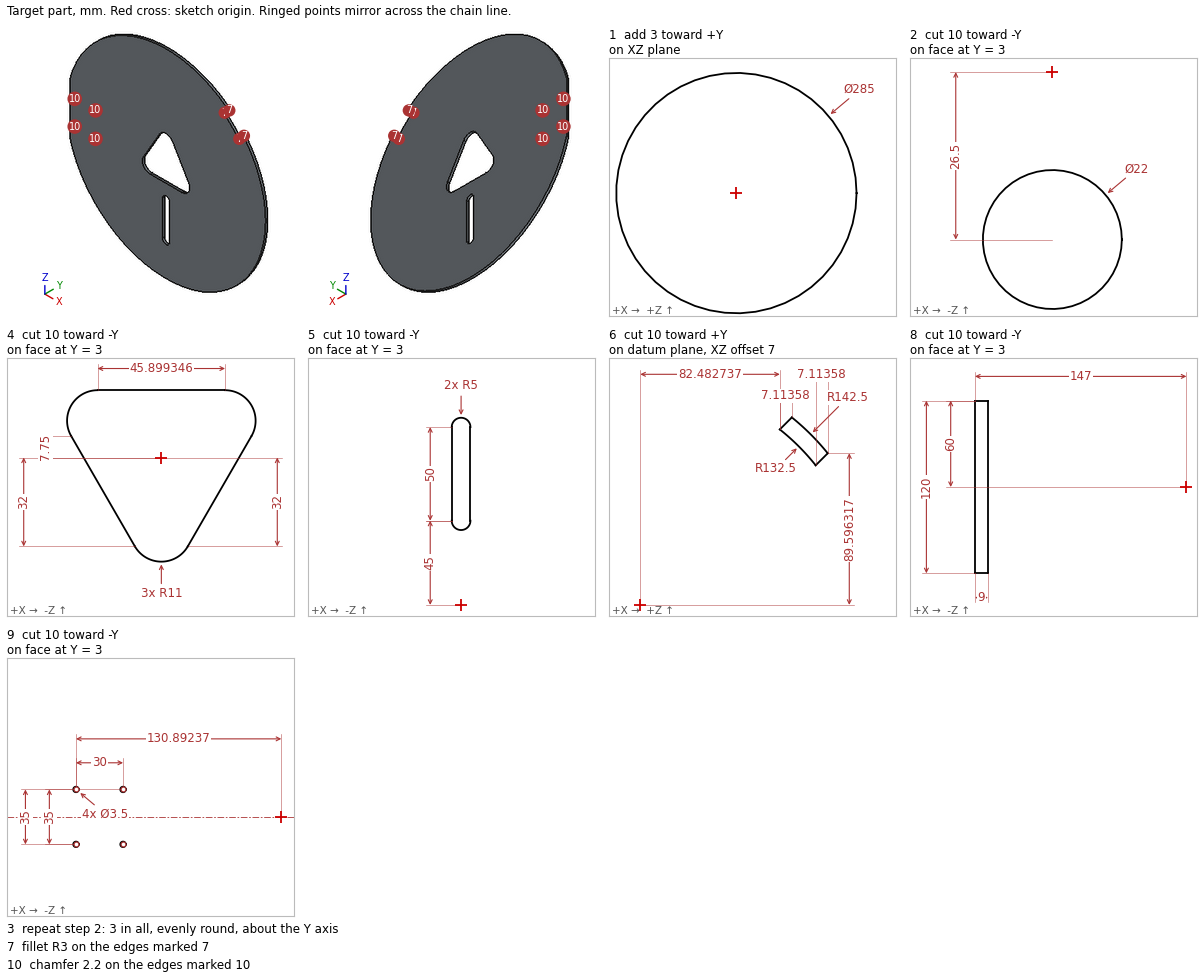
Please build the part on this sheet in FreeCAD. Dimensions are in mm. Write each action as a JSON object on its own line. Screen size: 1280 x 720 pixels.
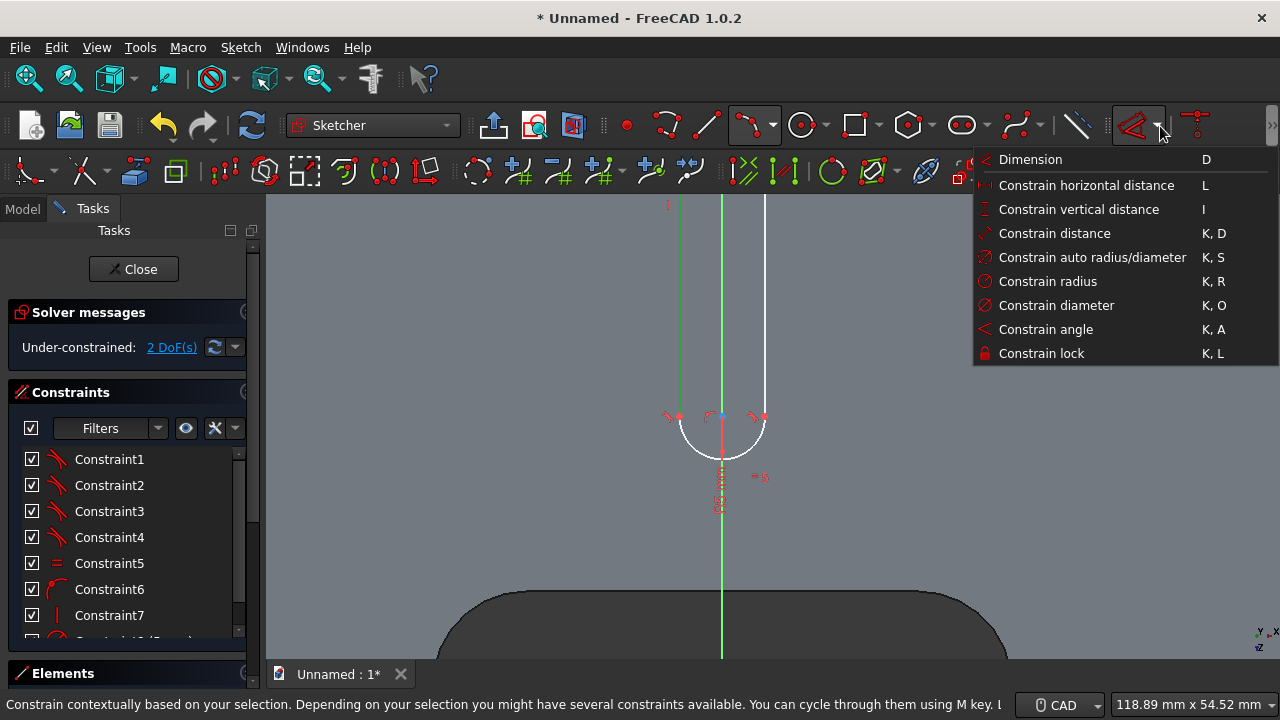
{"action": "left_click", "coordinate": [1126, 209]}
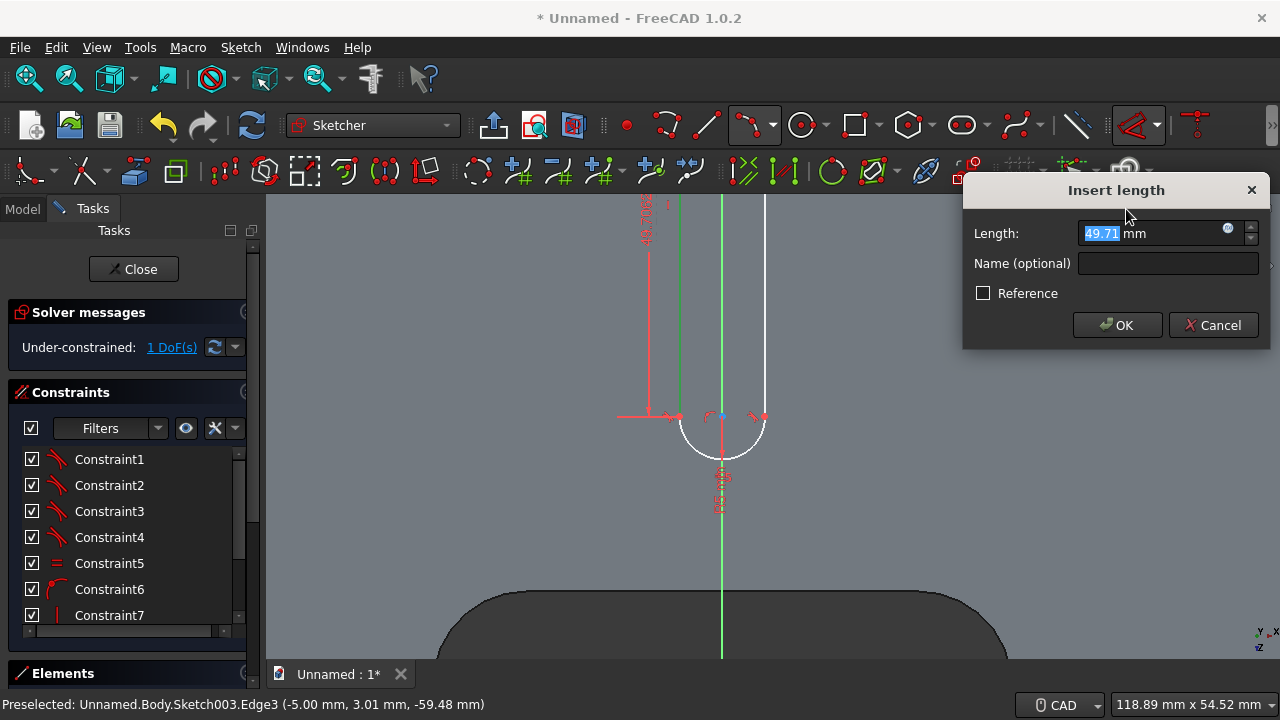
{"action": "type", "text": "50"}
{"action": "key", "text": "Return"}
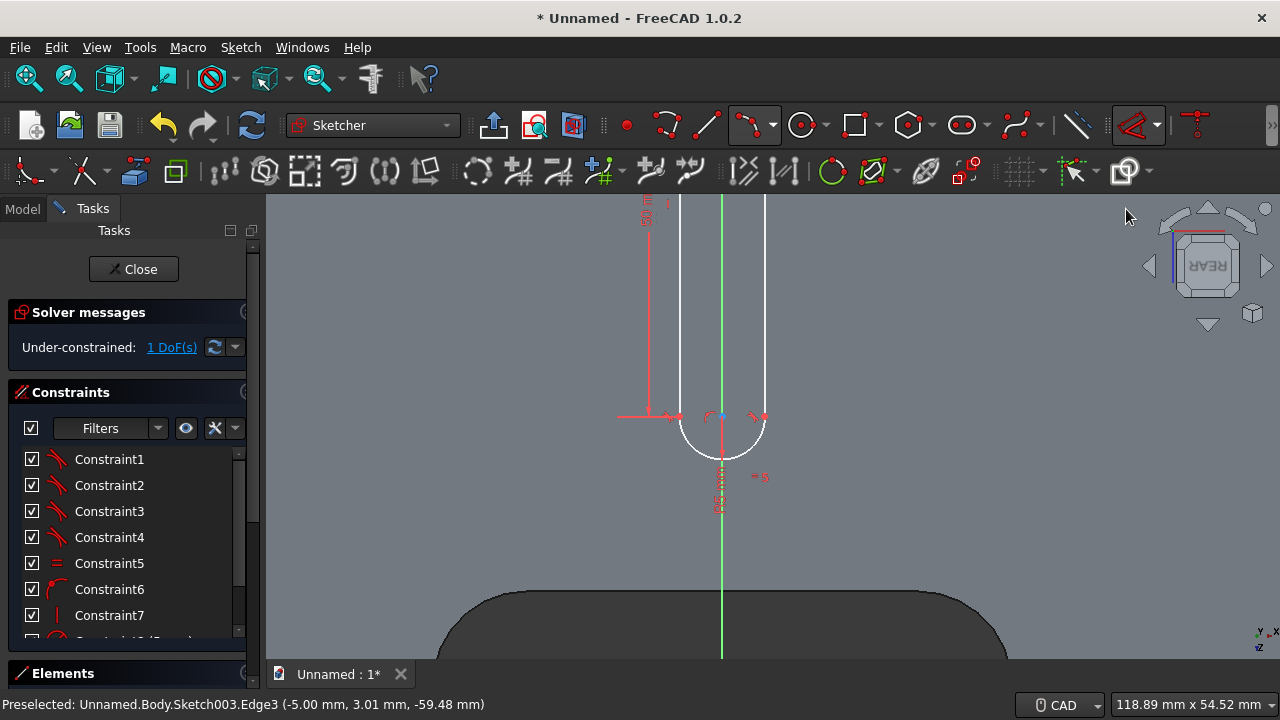
{"action": "left_click", "coordinate": [680, 417]}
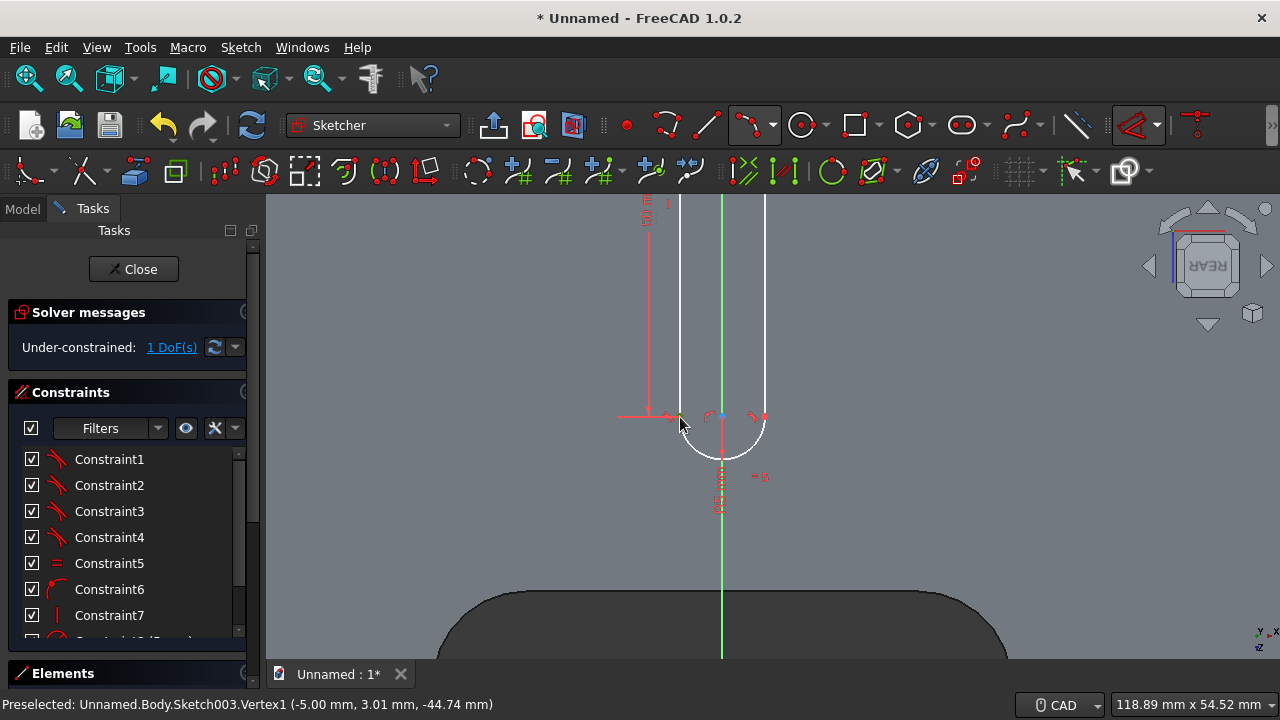
{"action": "key", "text": "i"}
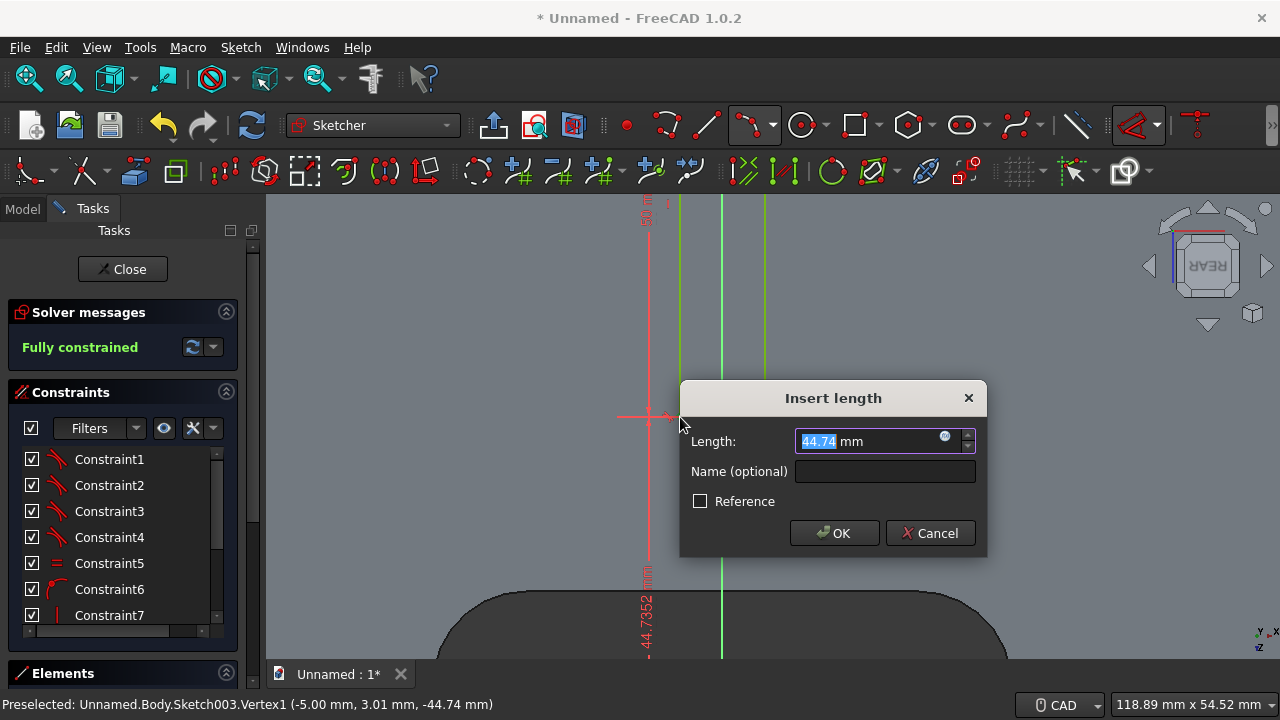
{"action": "type", "text": "45"}
{"action": "key", "text": "Return"}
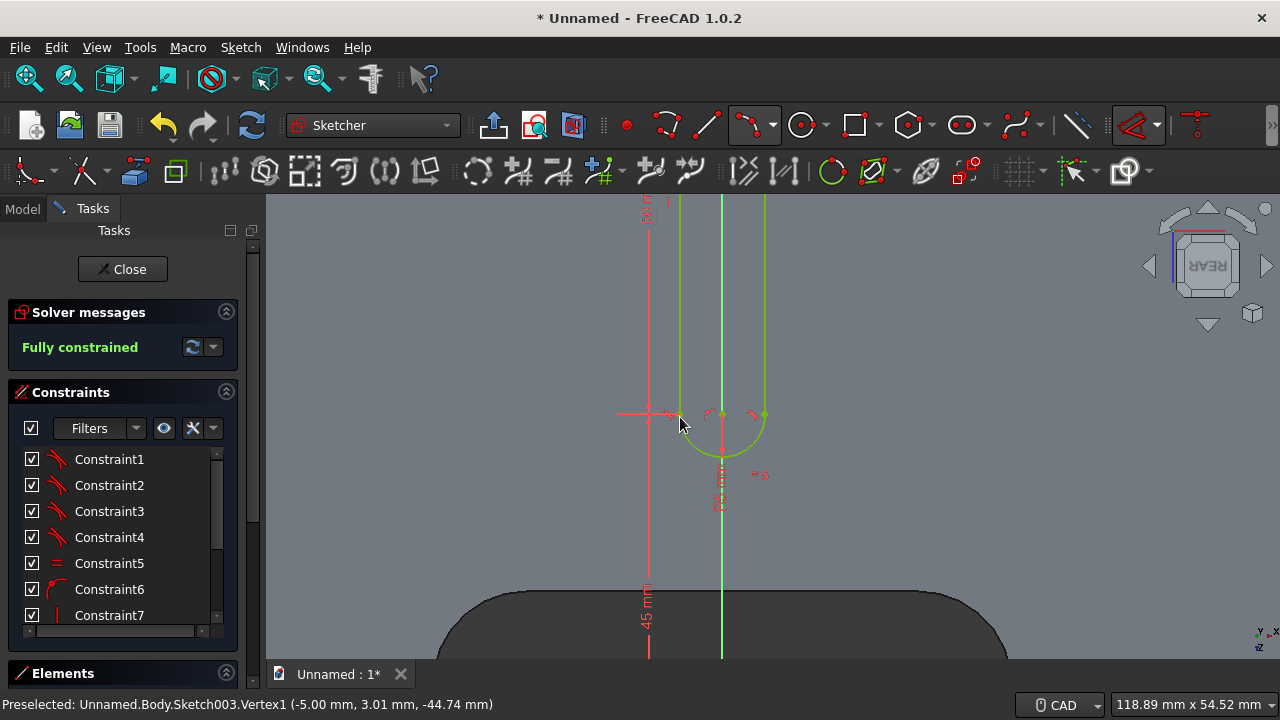
{"action": "left_click", "coordinate": [123, 269]}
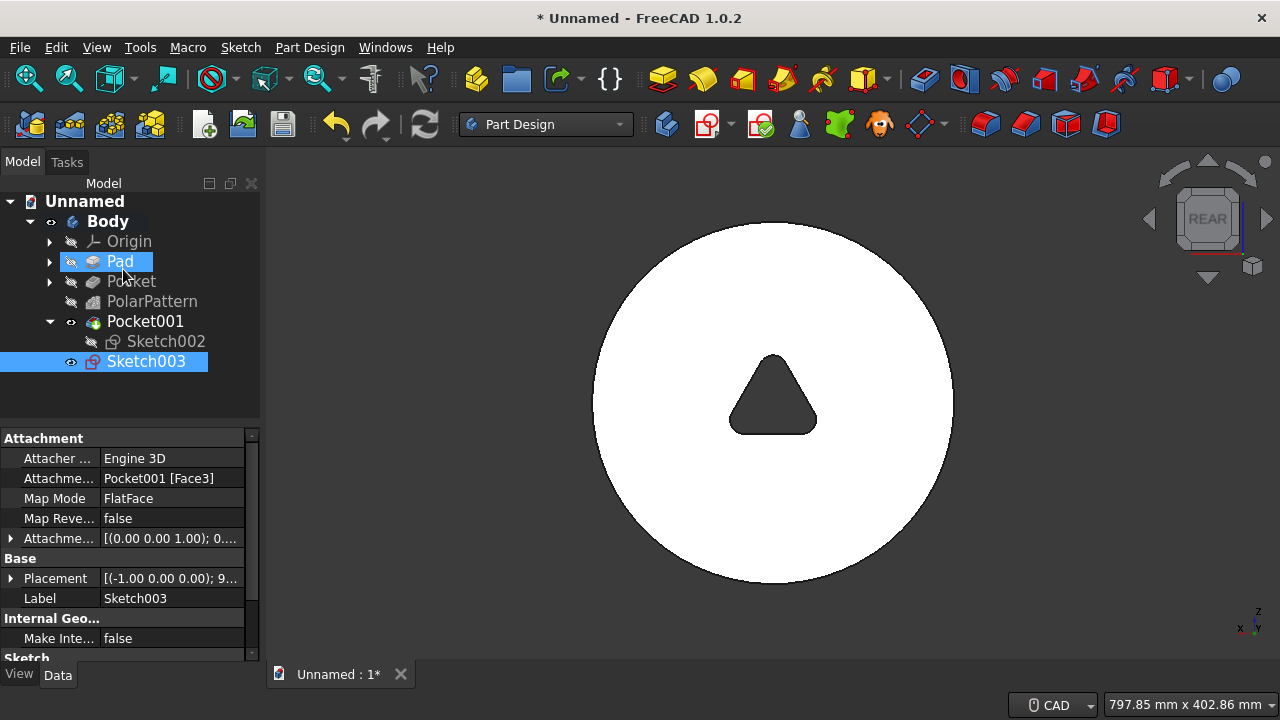
{"action": "left_click", "coordinate": [926, 80]}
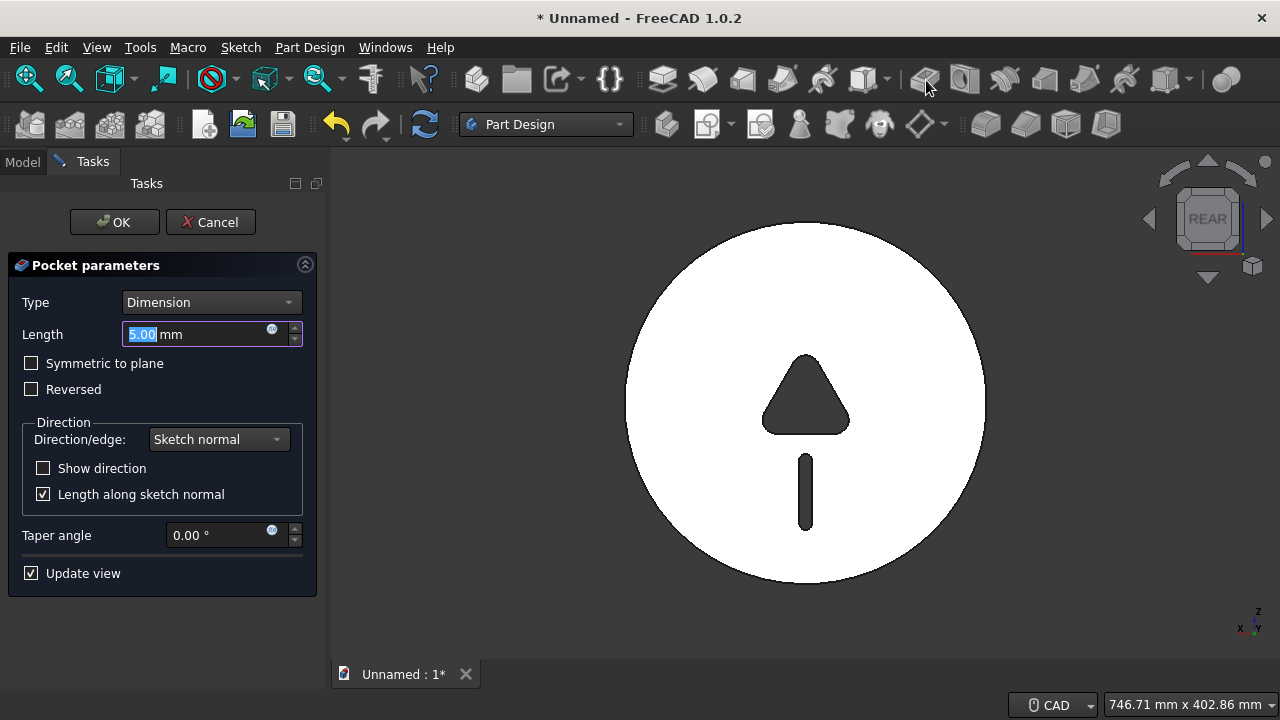
{"action": "type", "text": "10"}
{"action": "key", "text": "Tab"}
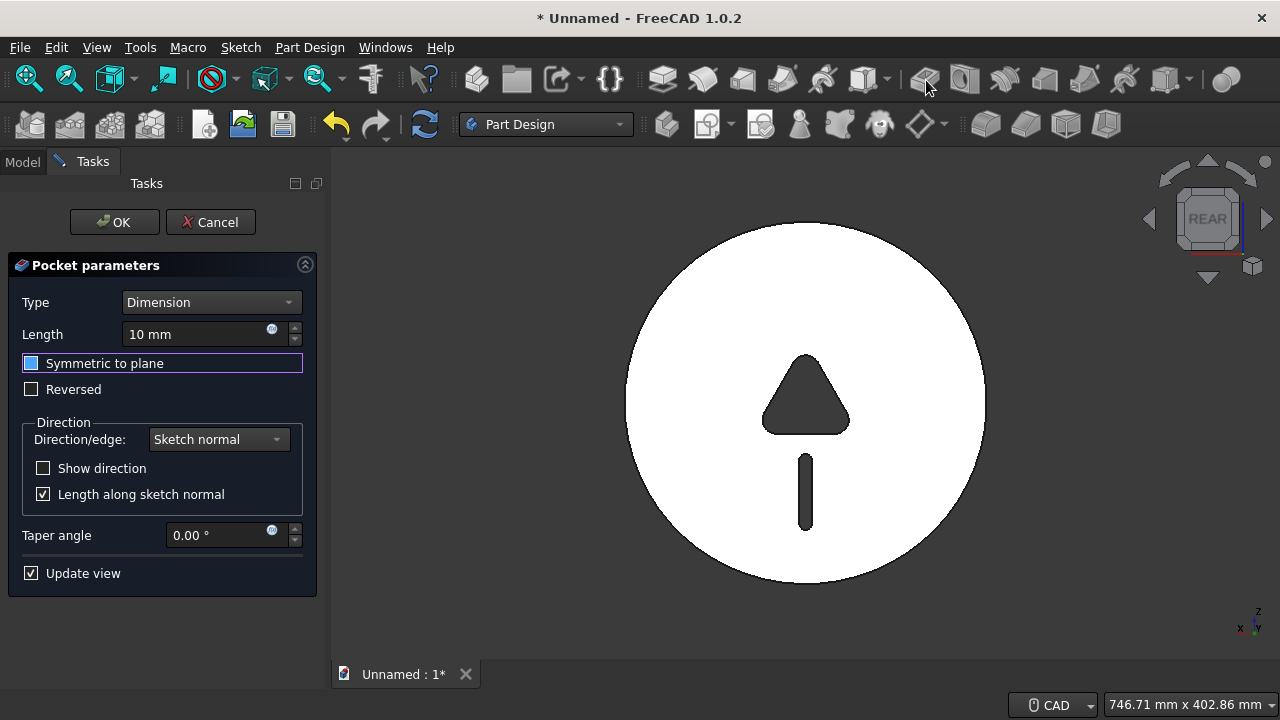
{"action": "left_click", "coordinate": [115, 222]}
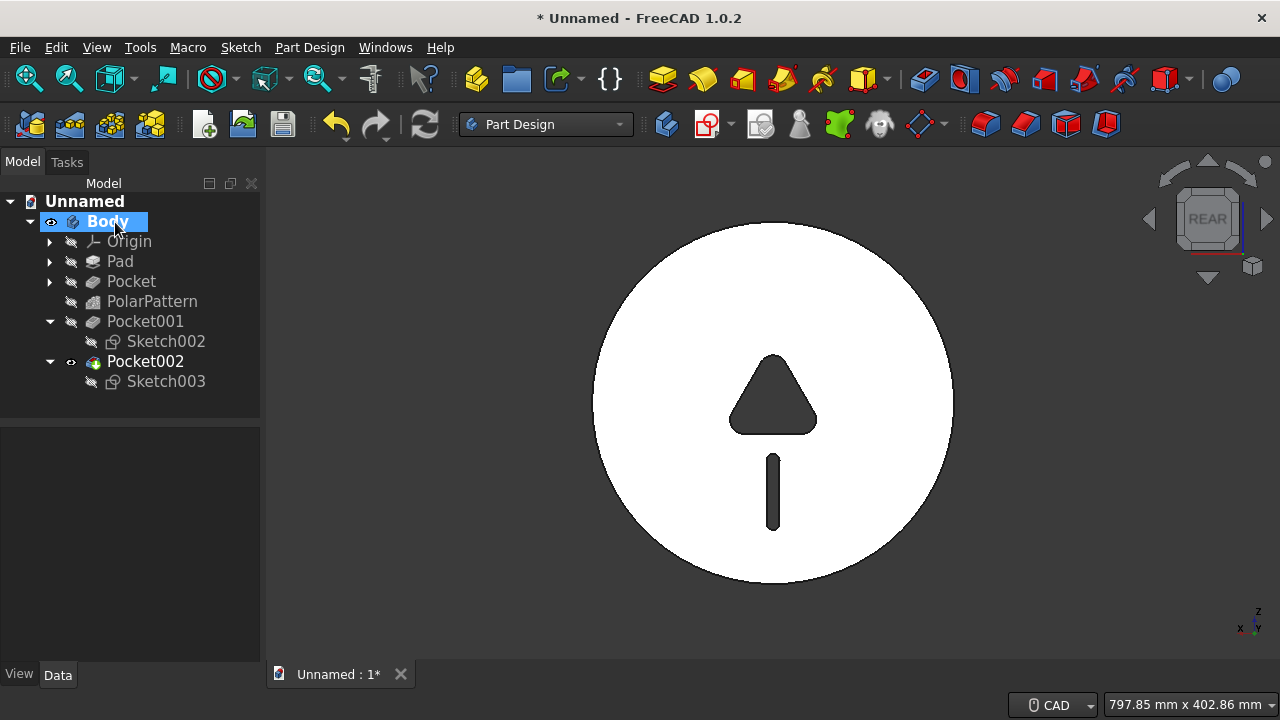
{"action": "left_click", "coordinate": [50, 242]}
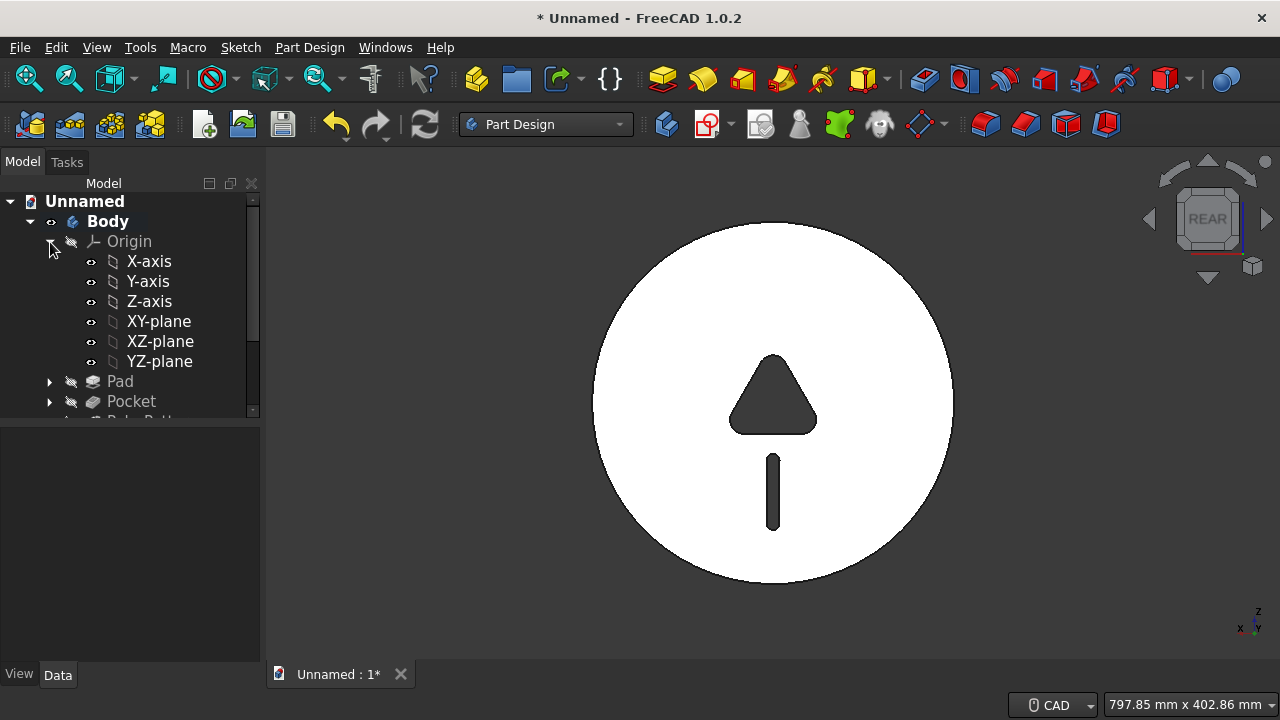
{"action": "left_click", "coordinate": [136, 342]}